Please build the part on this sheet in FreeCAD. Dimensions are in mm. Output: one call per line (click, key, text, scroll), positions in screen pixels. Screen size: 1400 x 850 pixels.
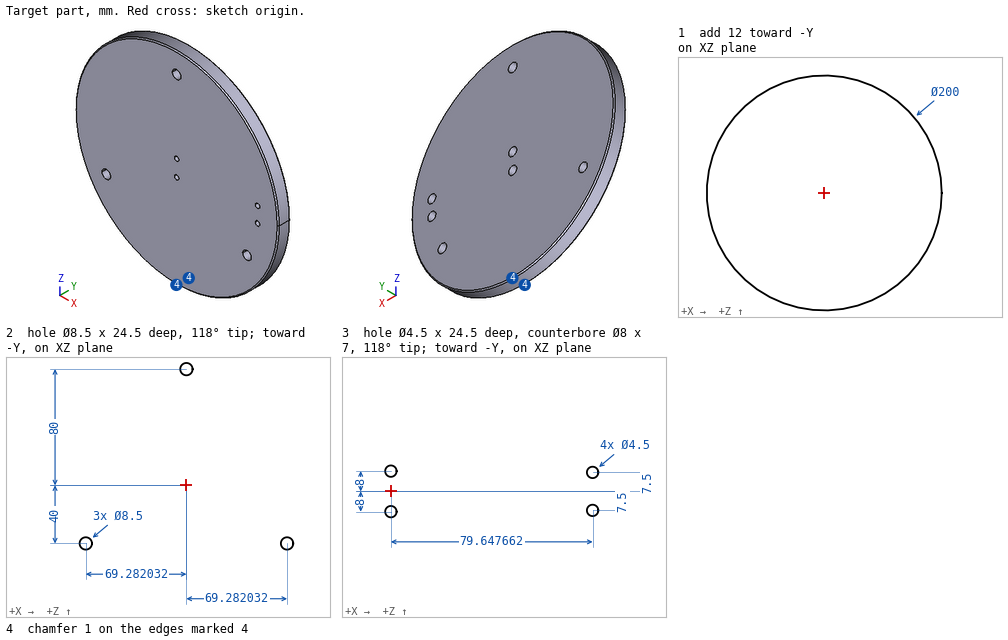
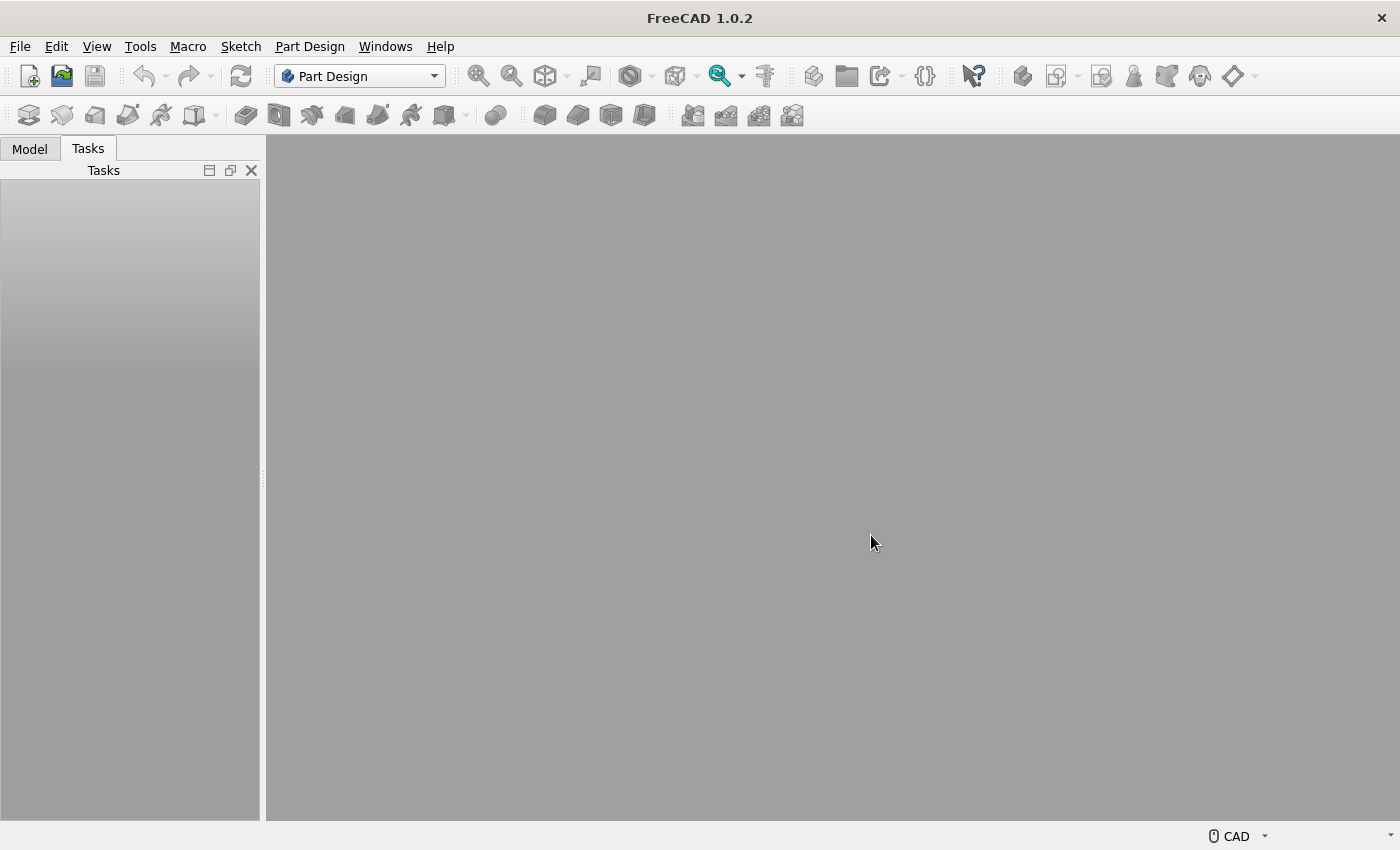
click(29, 76)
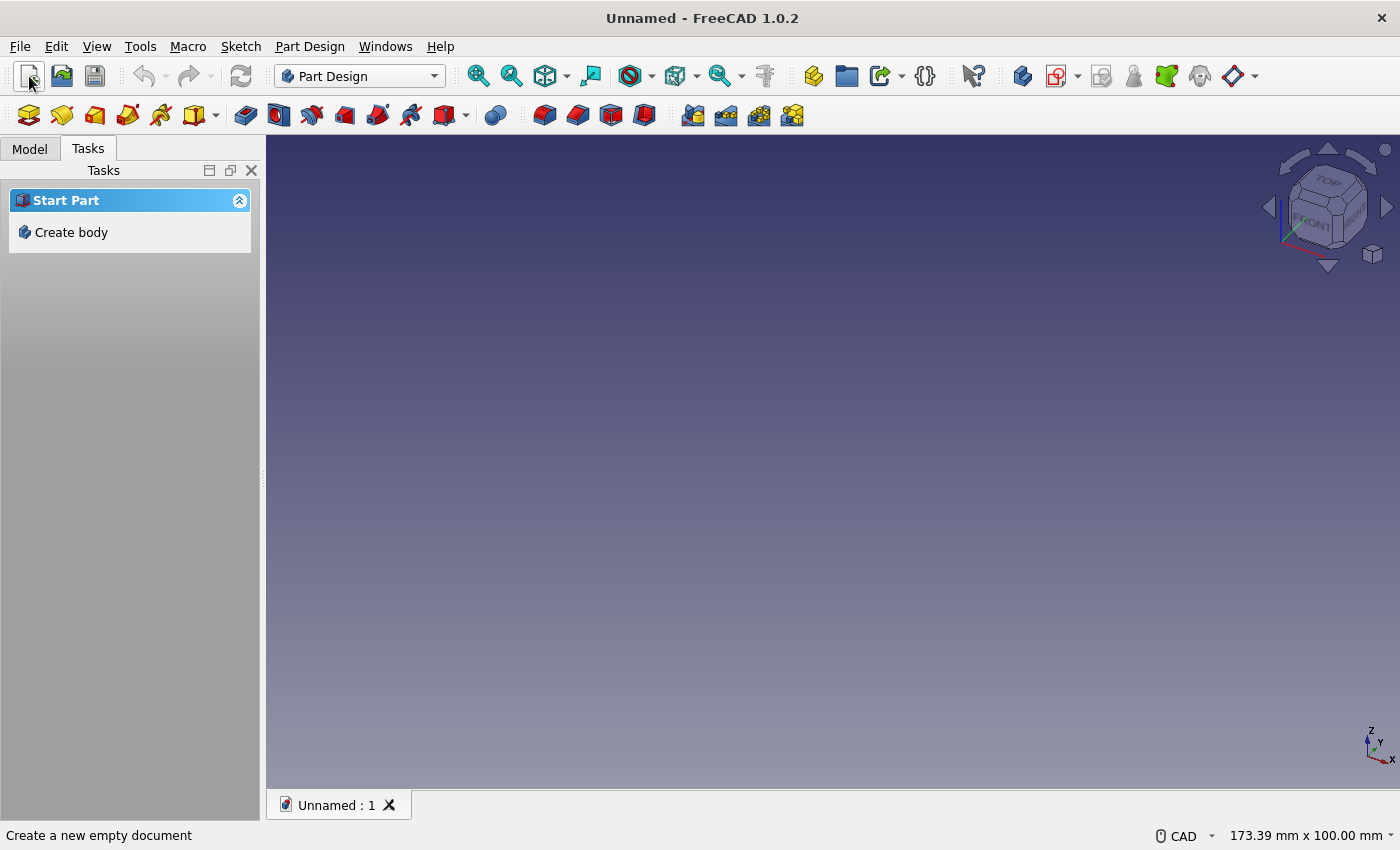
click(1056, 76)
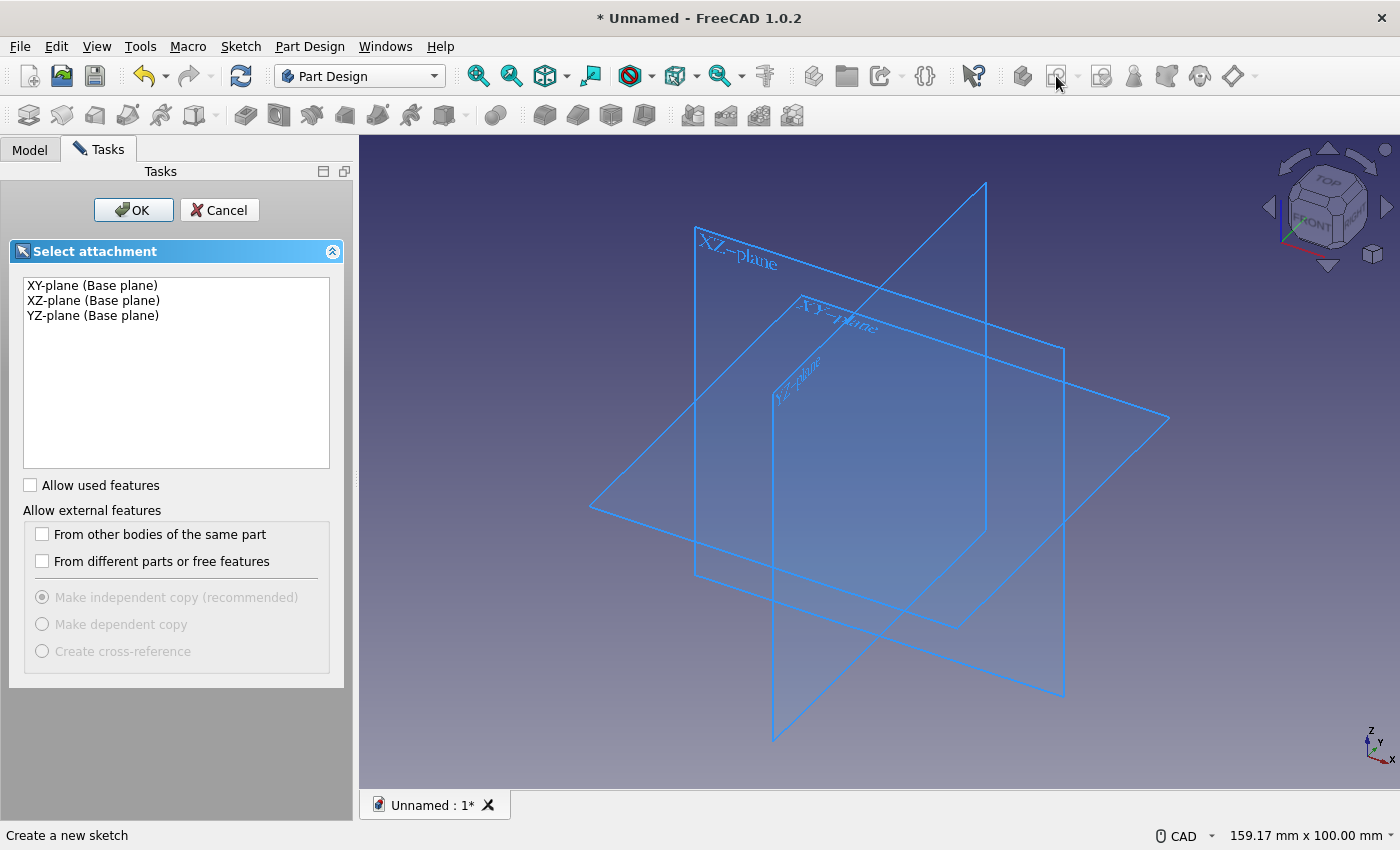
click(84, 300)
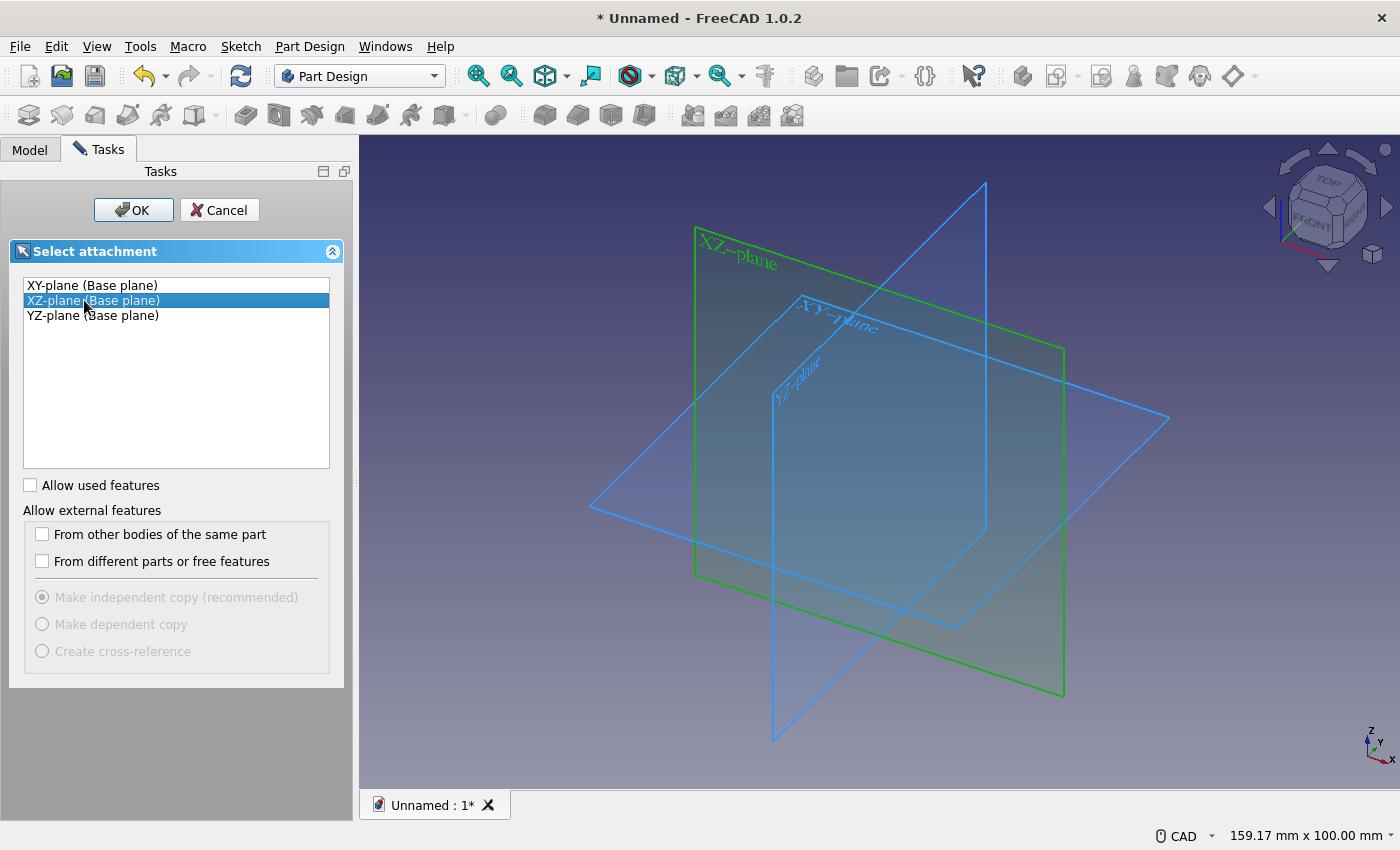
click(134, 210)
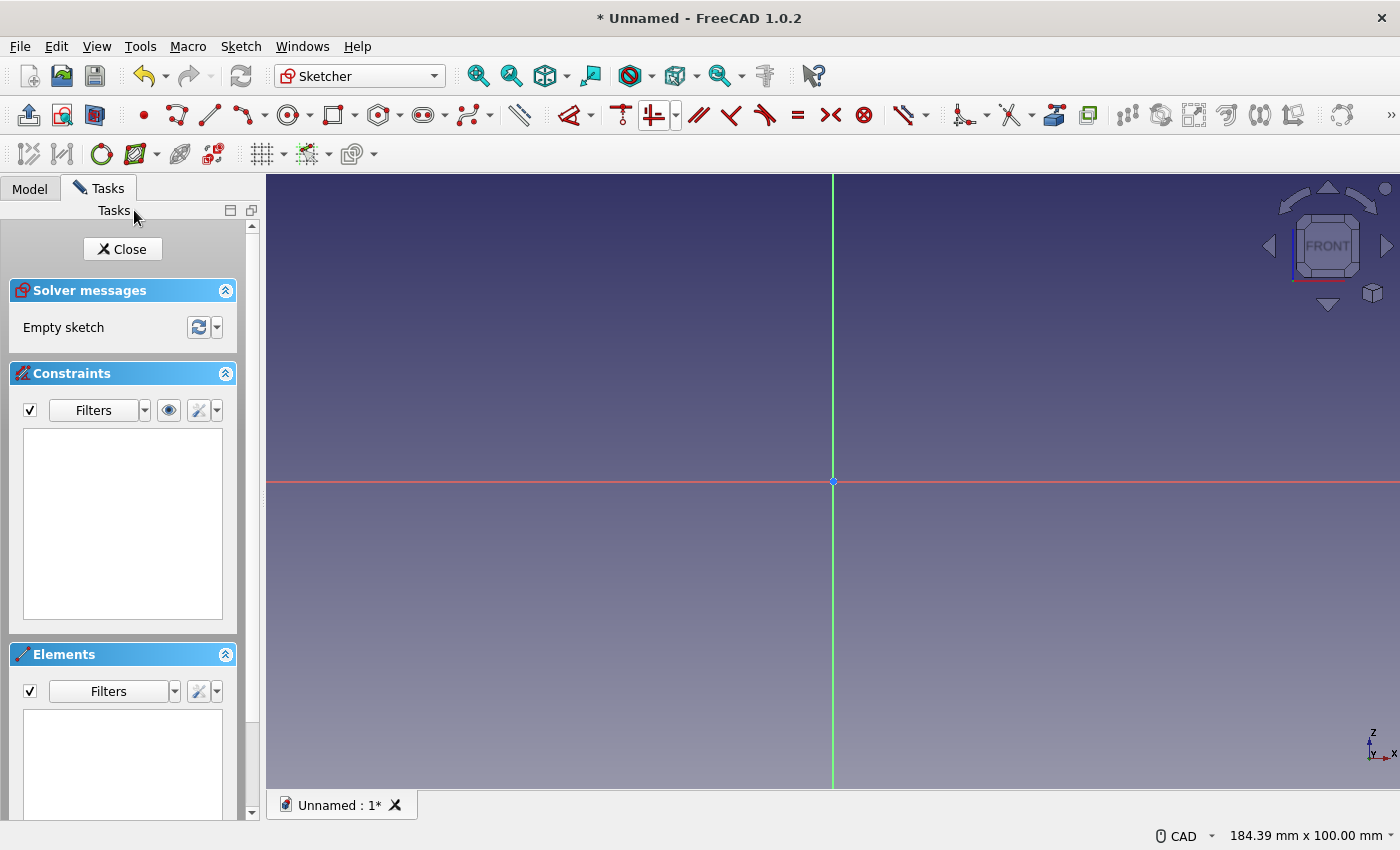
scroll(735, 481, down, 6)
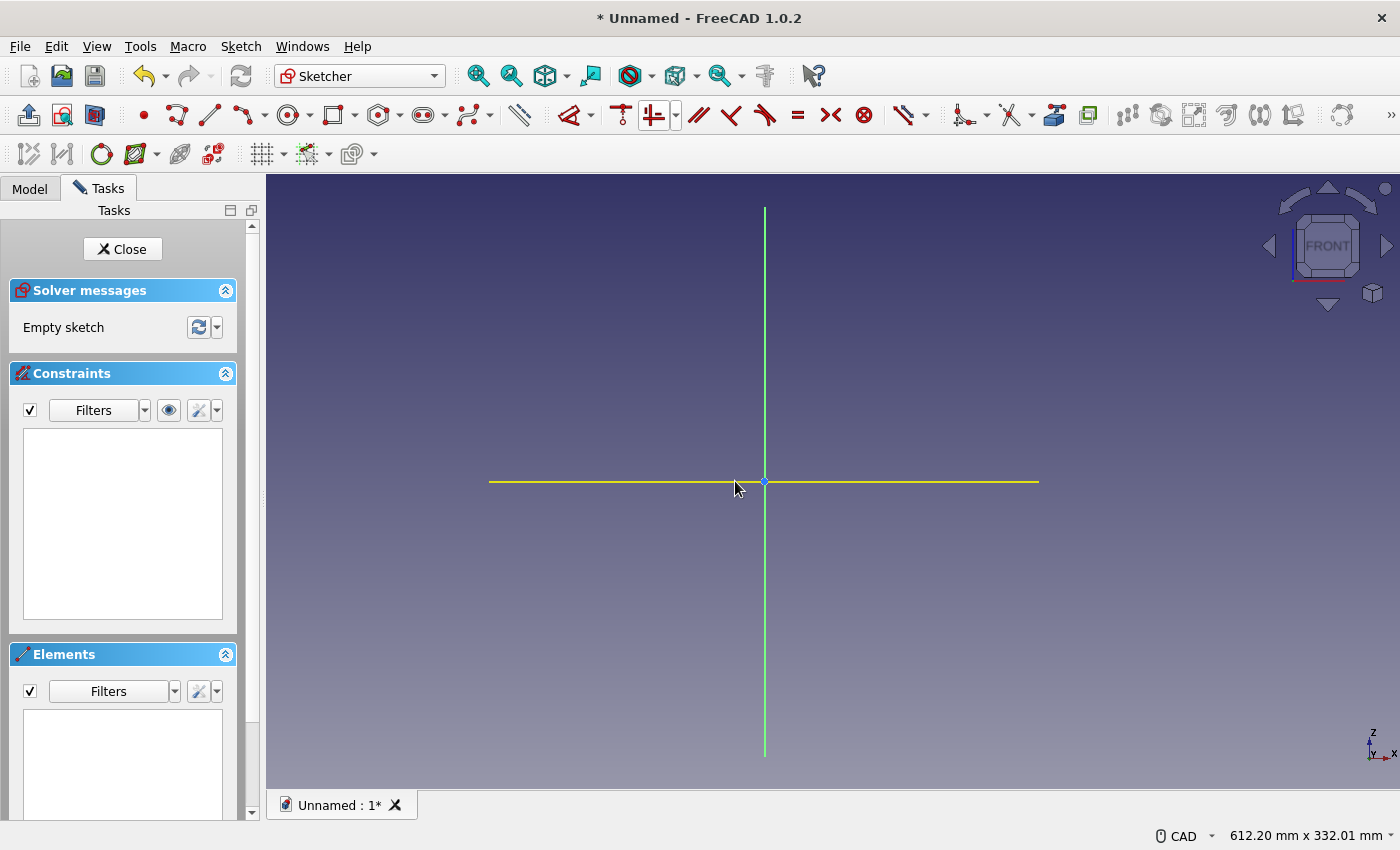
key(g)
key(c)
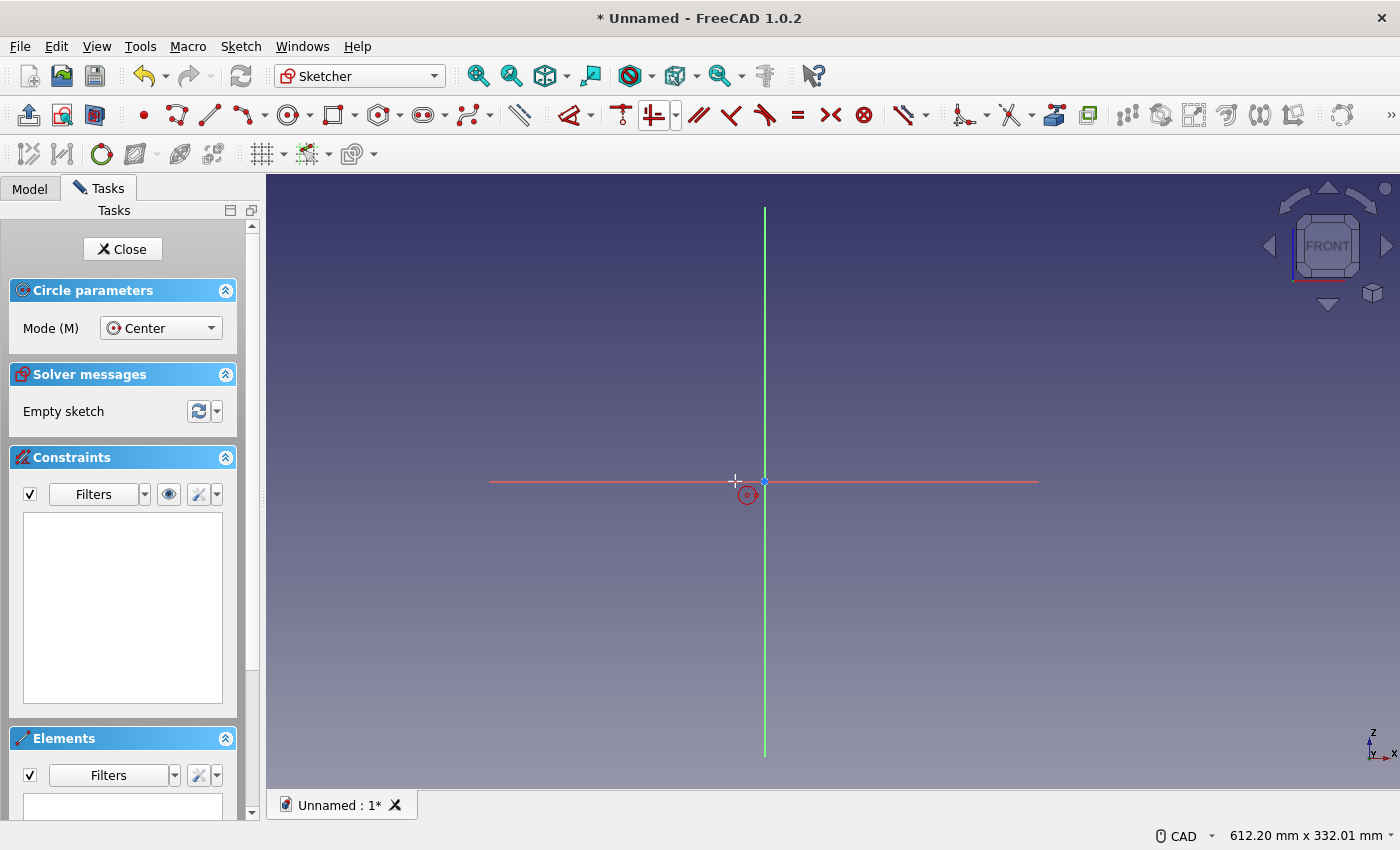
click(765, 482)
move(896, 351)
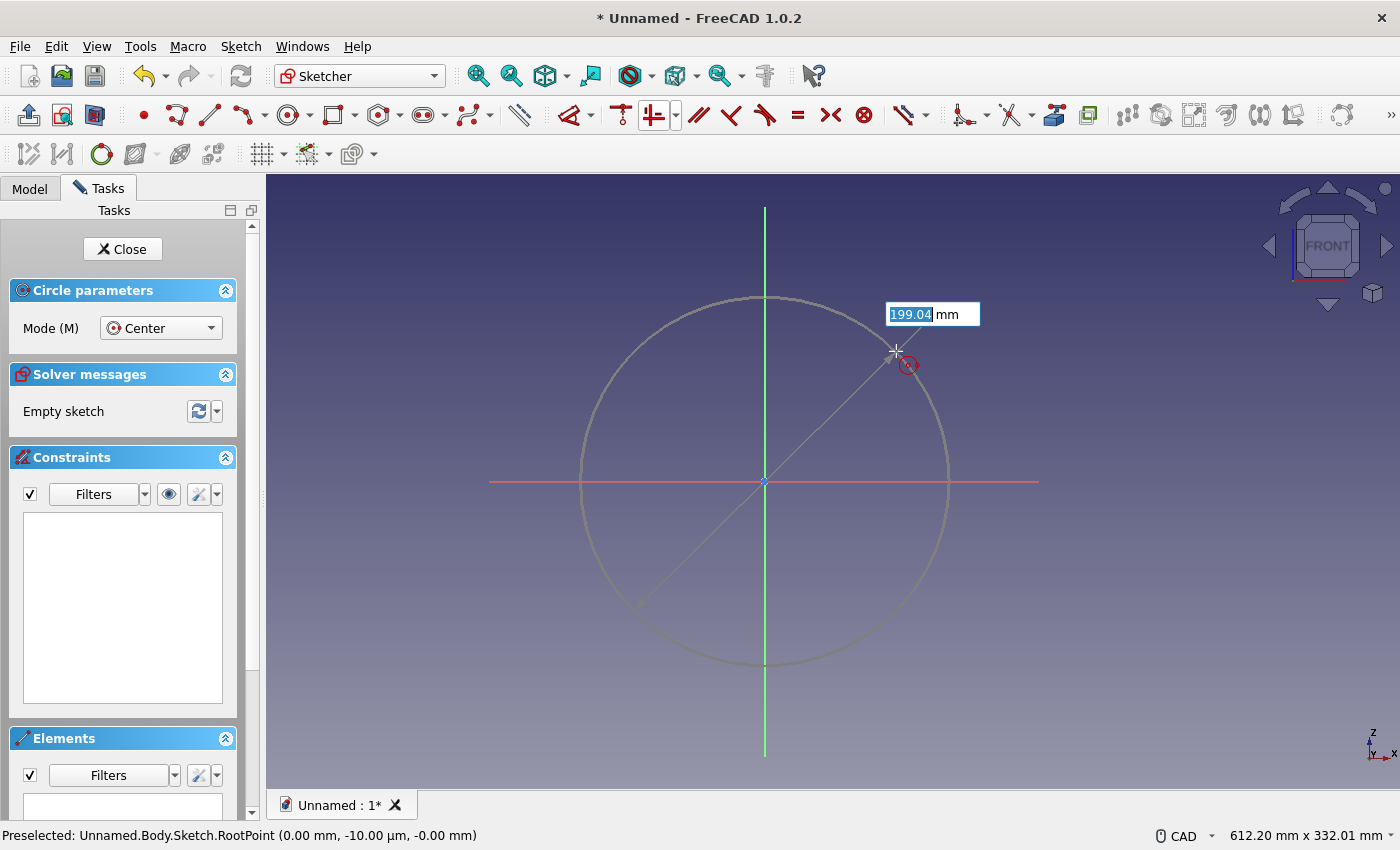
text(200)
key(Return)
key(Escape)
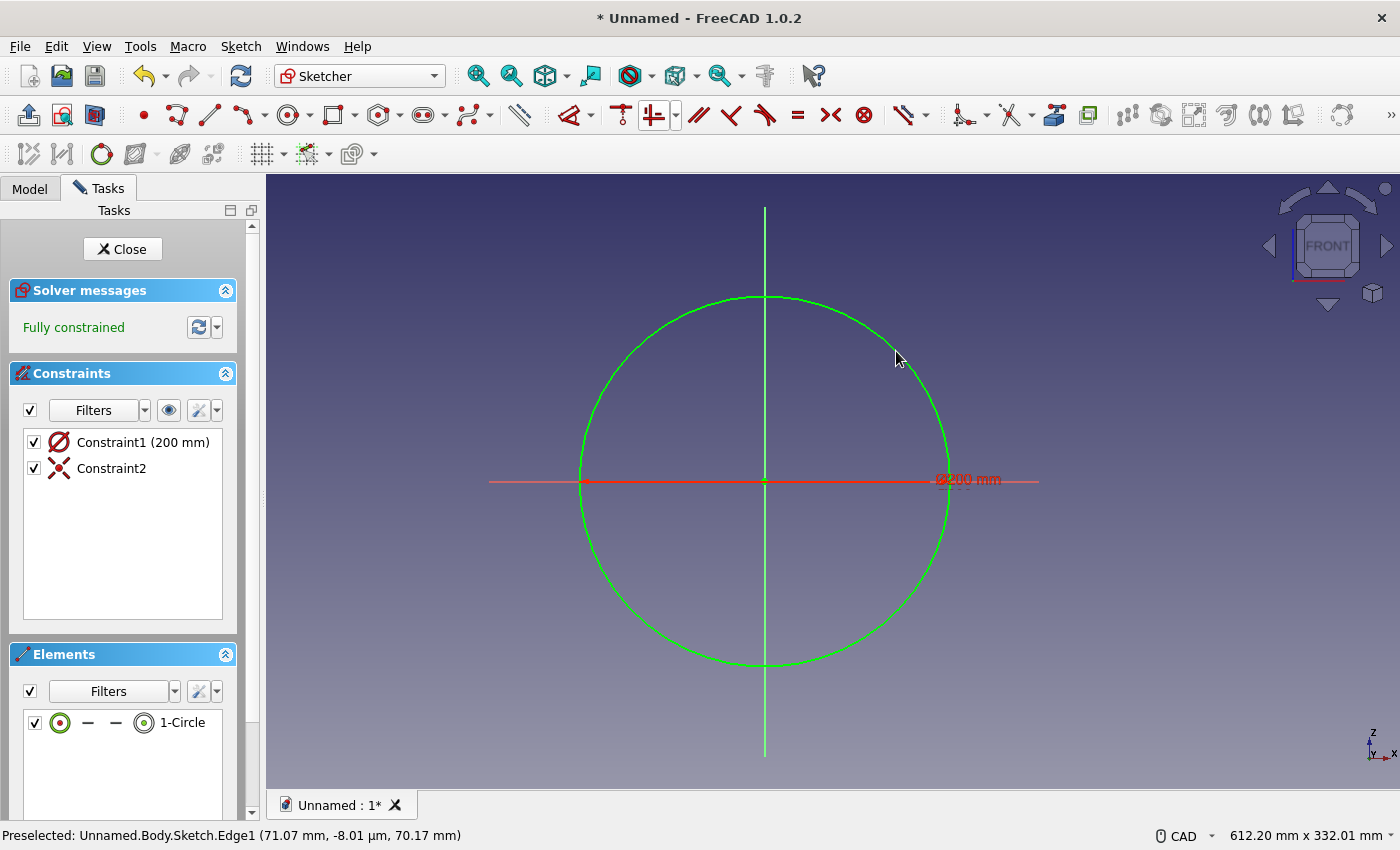
click(123, 249)